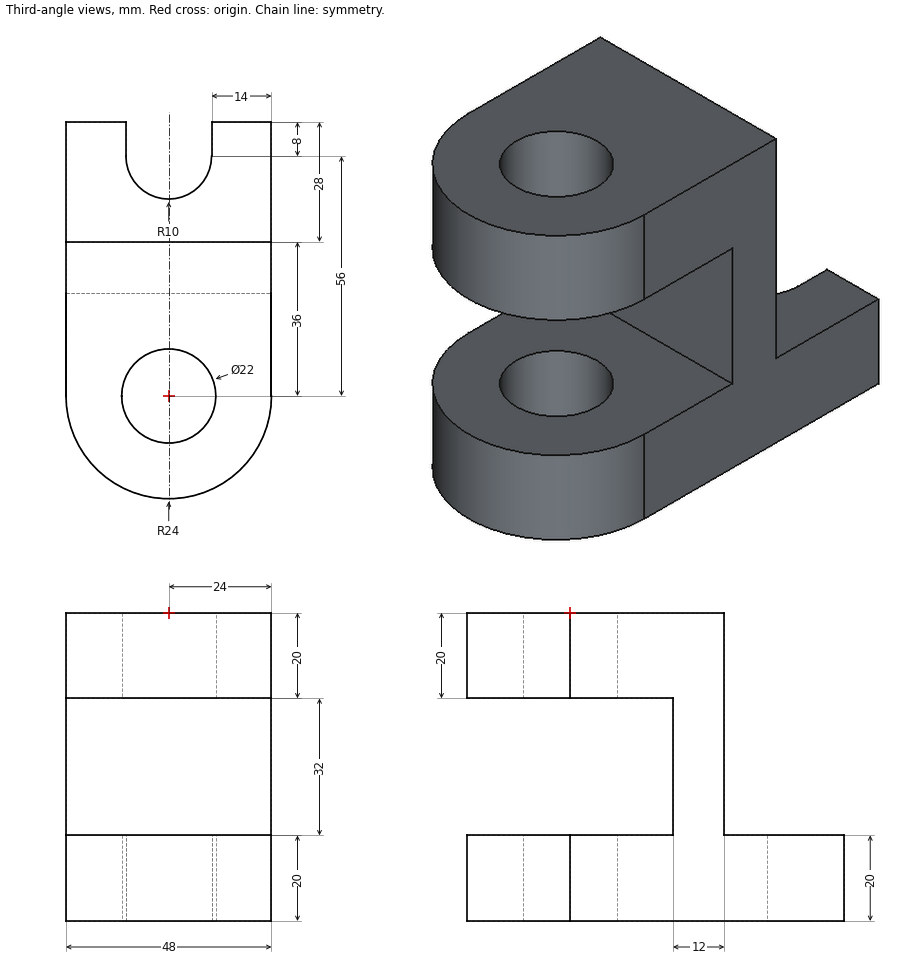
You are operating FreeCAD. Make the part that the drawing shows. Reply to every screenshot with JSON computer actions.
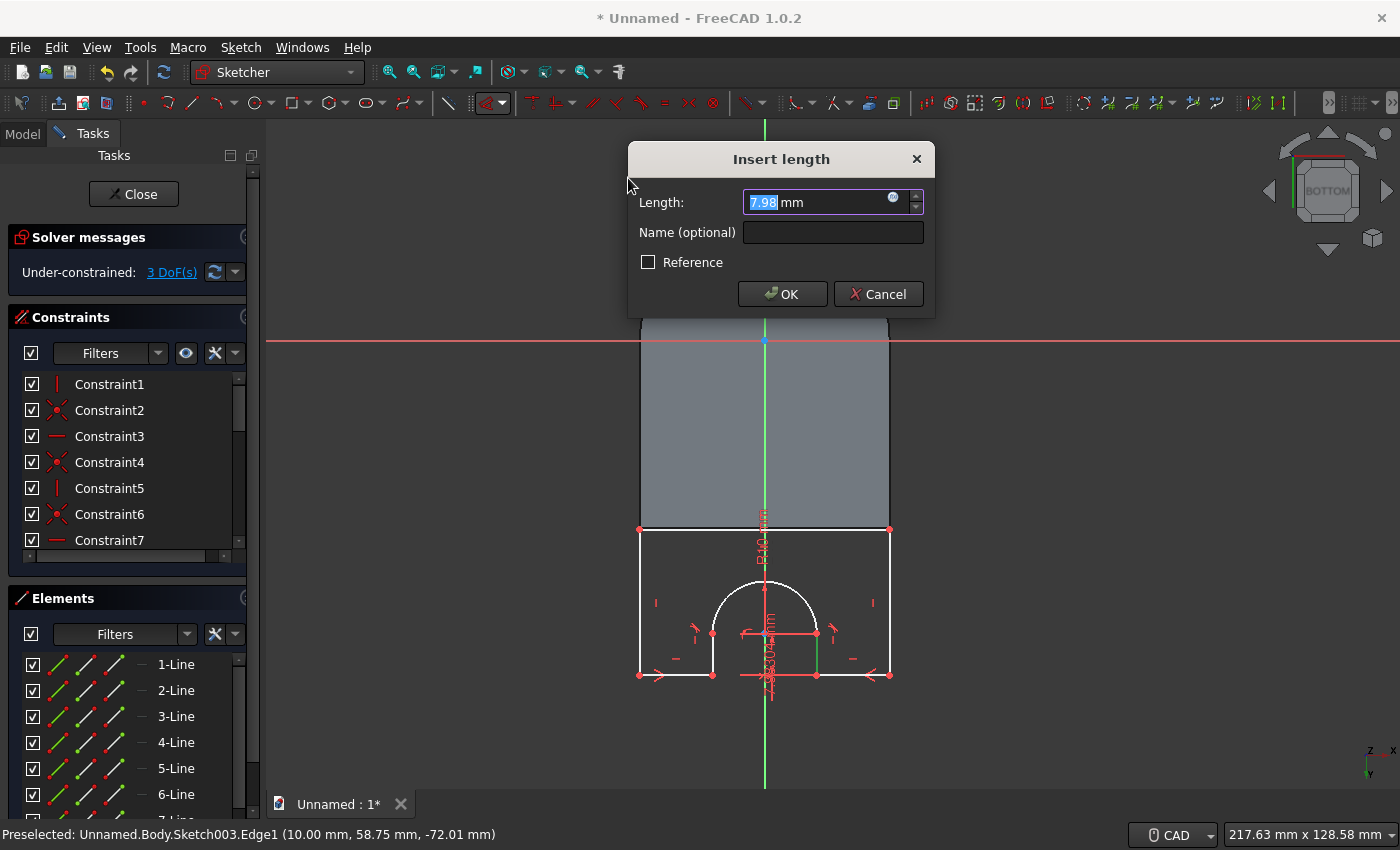
{"action": "type", "text": "8"}
{"action": "key", "text": "Return"}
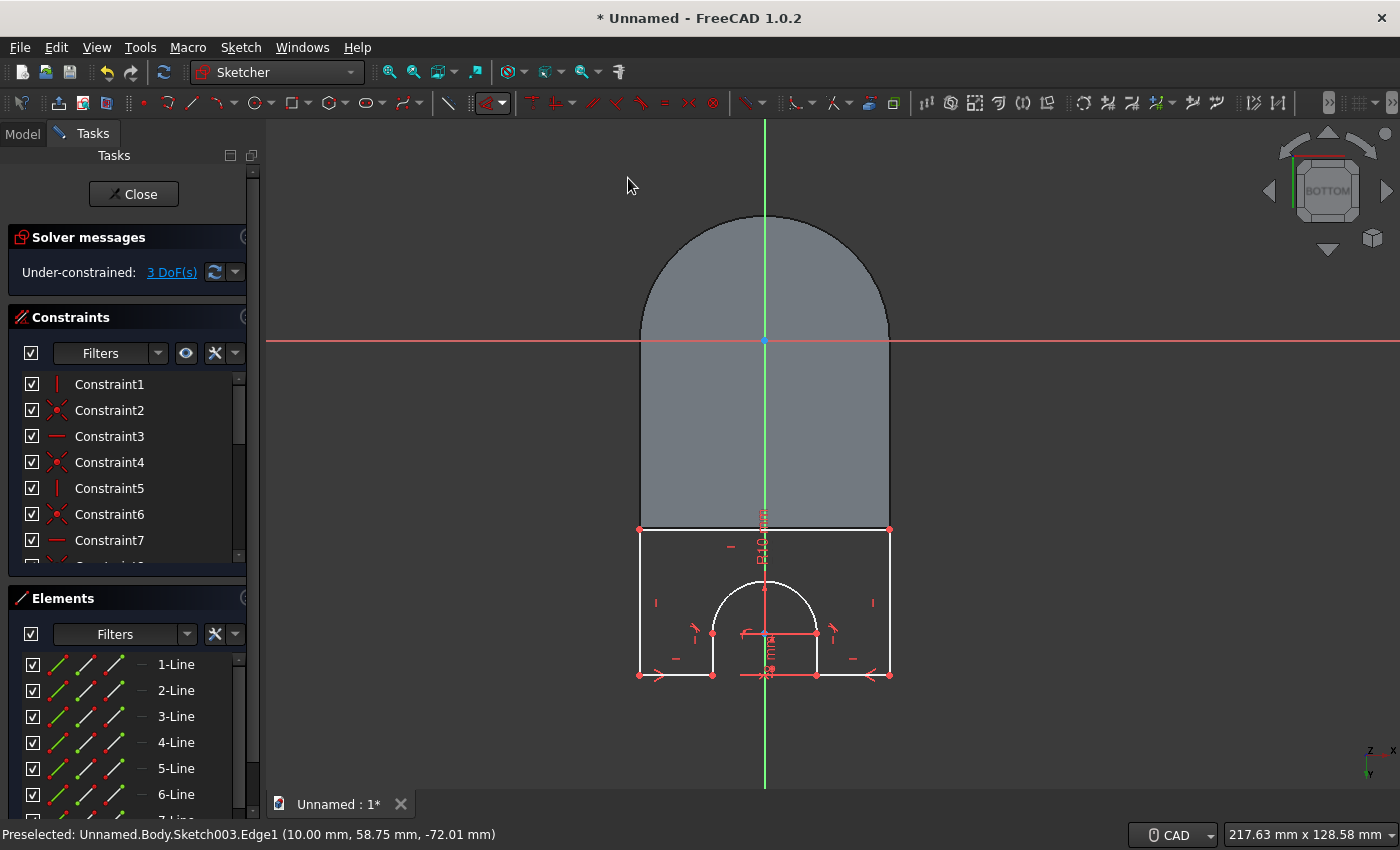
{"action": "left_click", "coordinate": [839, 675]}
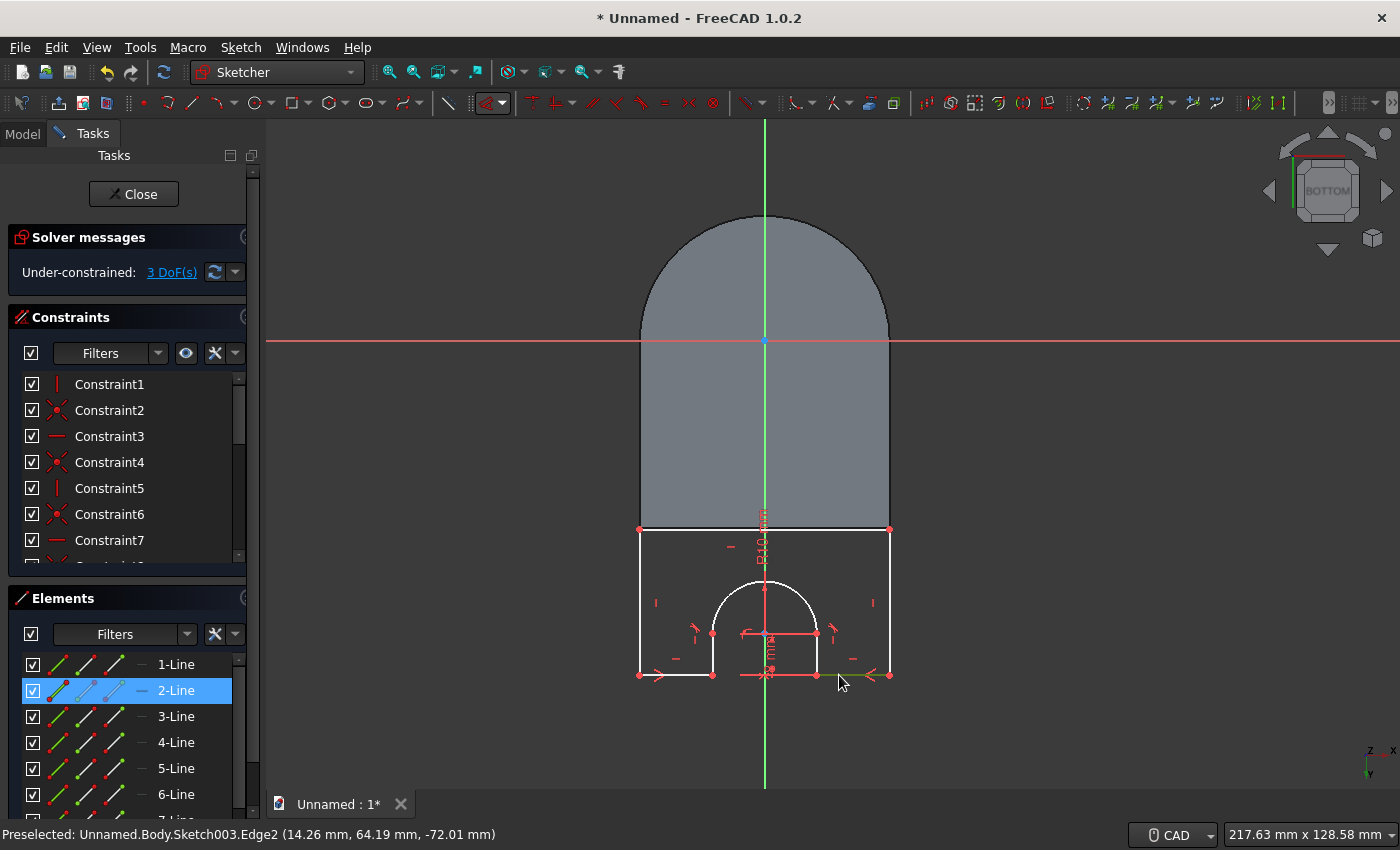
{"action": "key", "text": "l"}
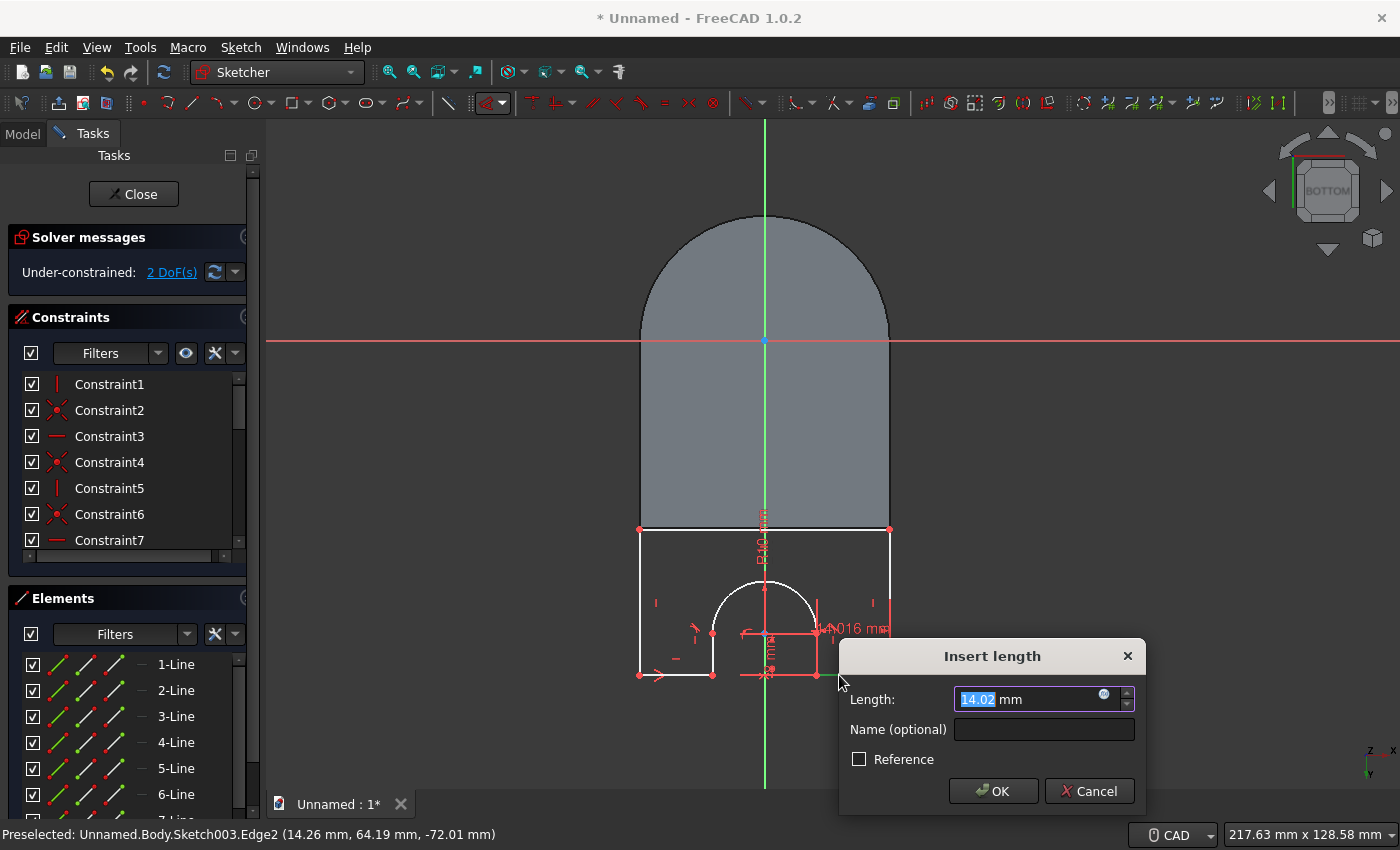
{"action": "type", "text": "14"}
{"action": "key", "text": "Return"}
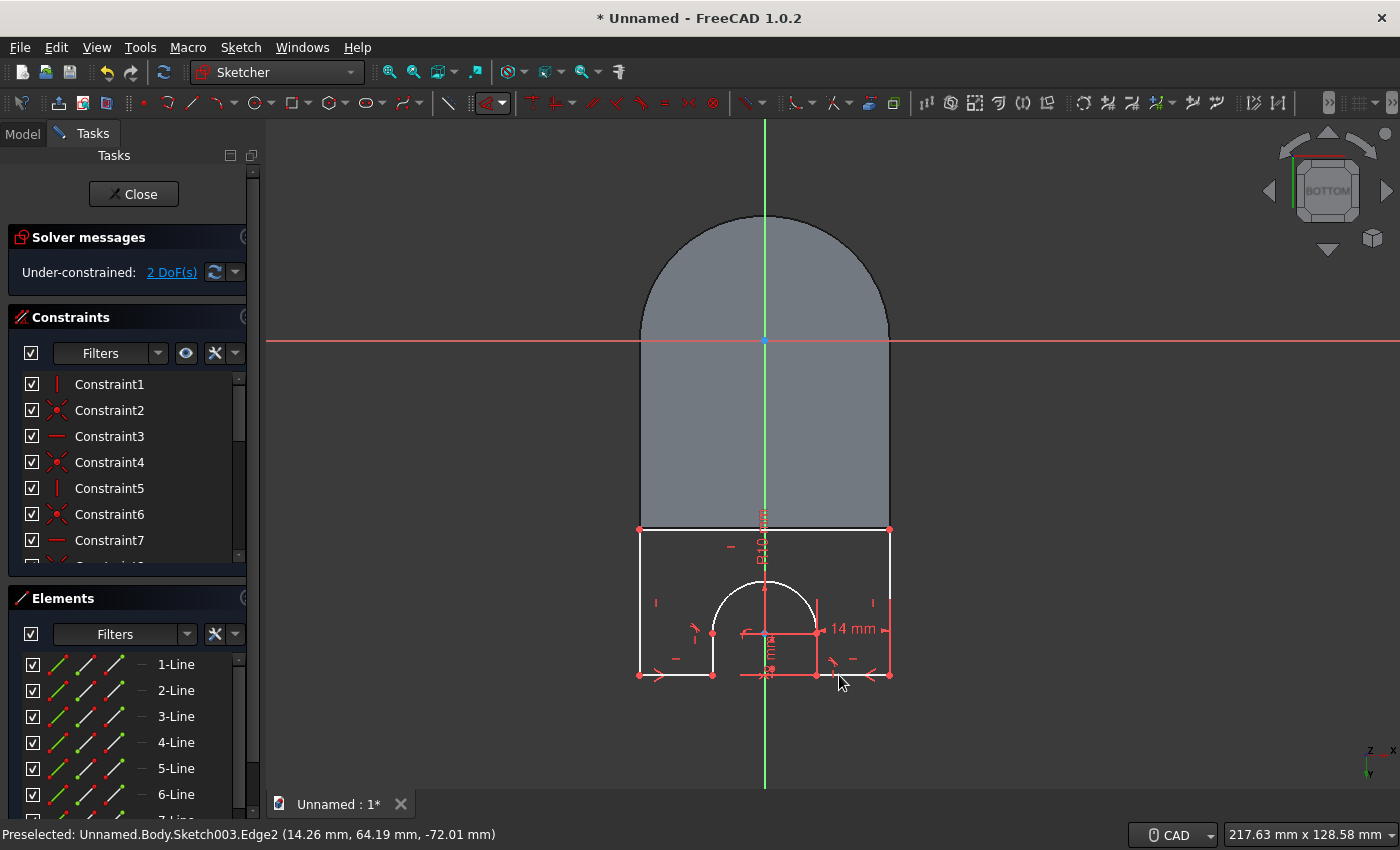
{"action": "left_click", "coordinate": [890, 632]}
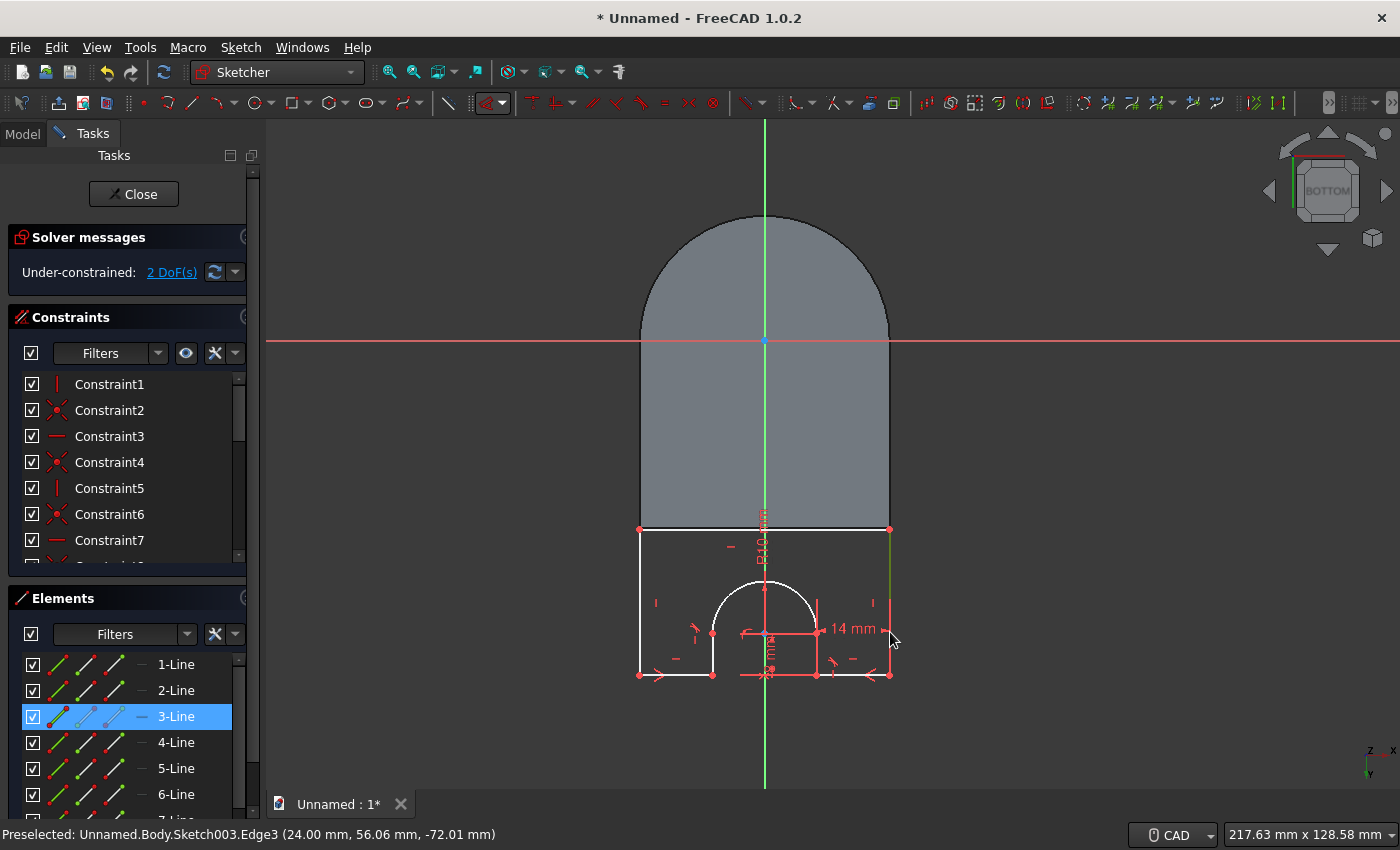
{"action": "key", "text": "i"}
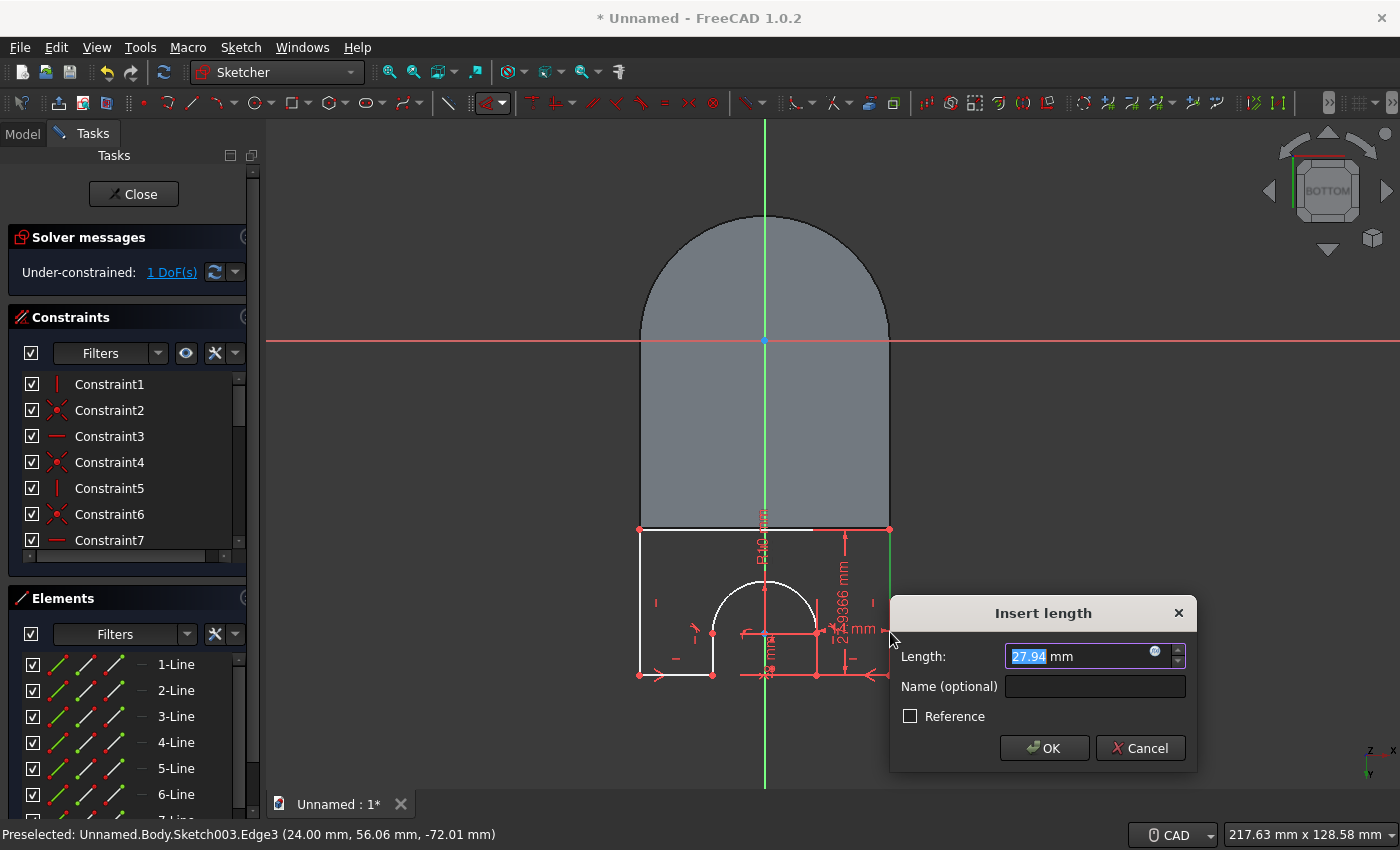
{"action": "type", "text": "28"}
{"action": "key", "text": "Return"}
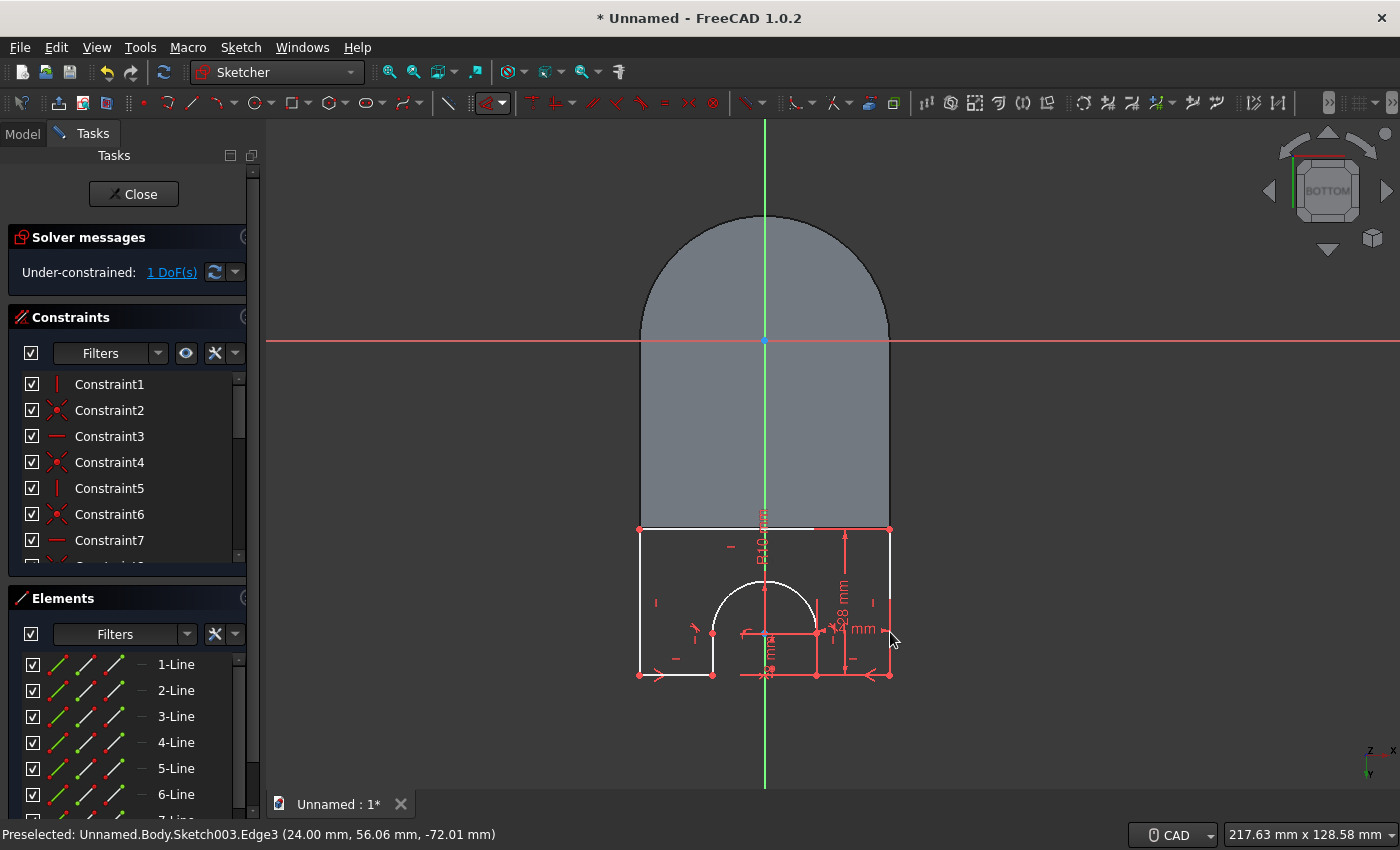
{"action": "left_click", "coordinate": [817, 634]}